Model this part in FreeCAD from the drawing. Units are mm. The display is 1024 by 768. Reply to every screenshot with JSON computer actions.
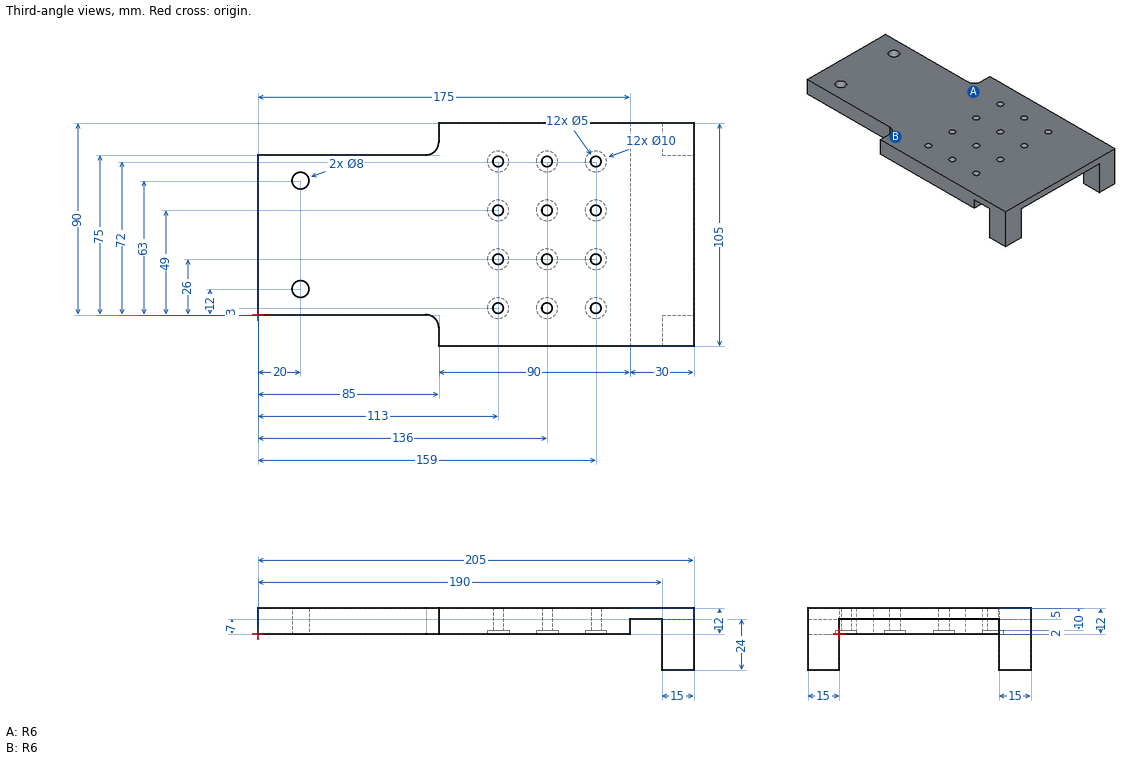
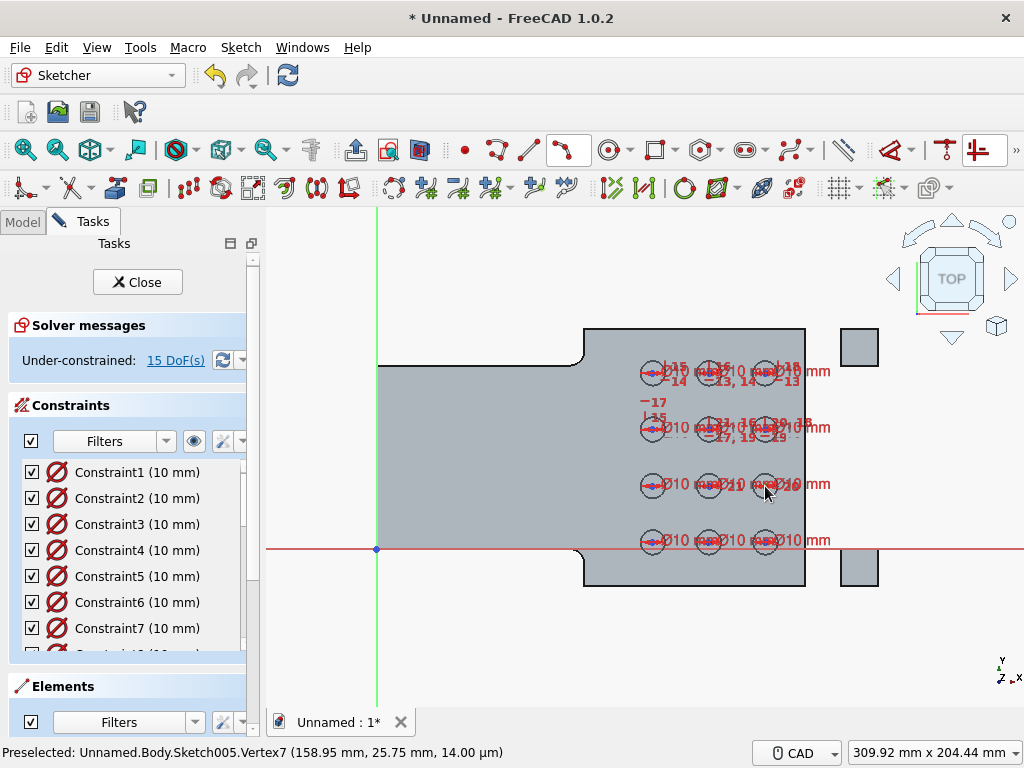
{"action": "left_click", "coordinate": [709, 486]}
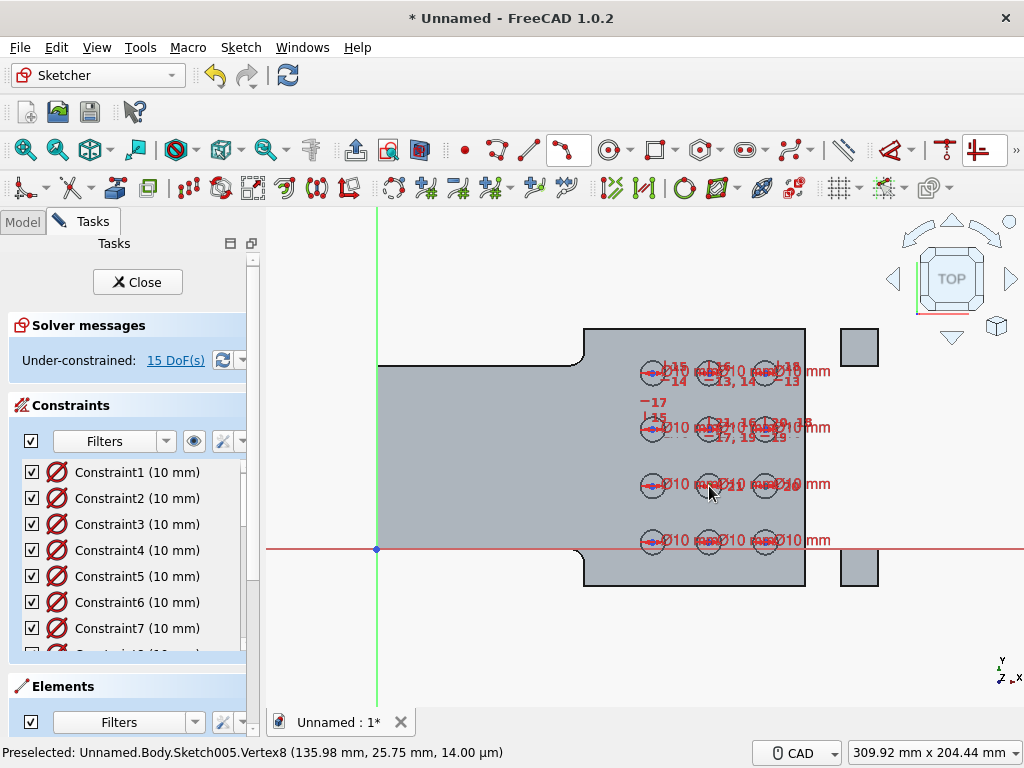
{"action": "left_click", "coordinate": [1002, 150]}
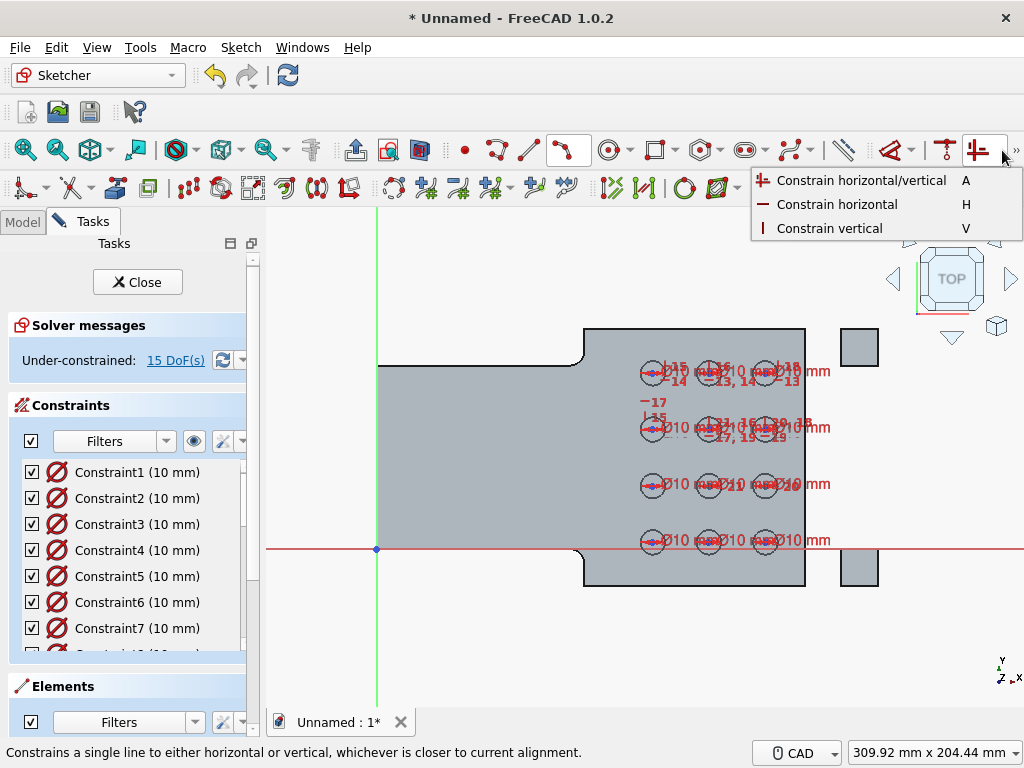
{"action": "left_click", "coordinate": [887, 204]}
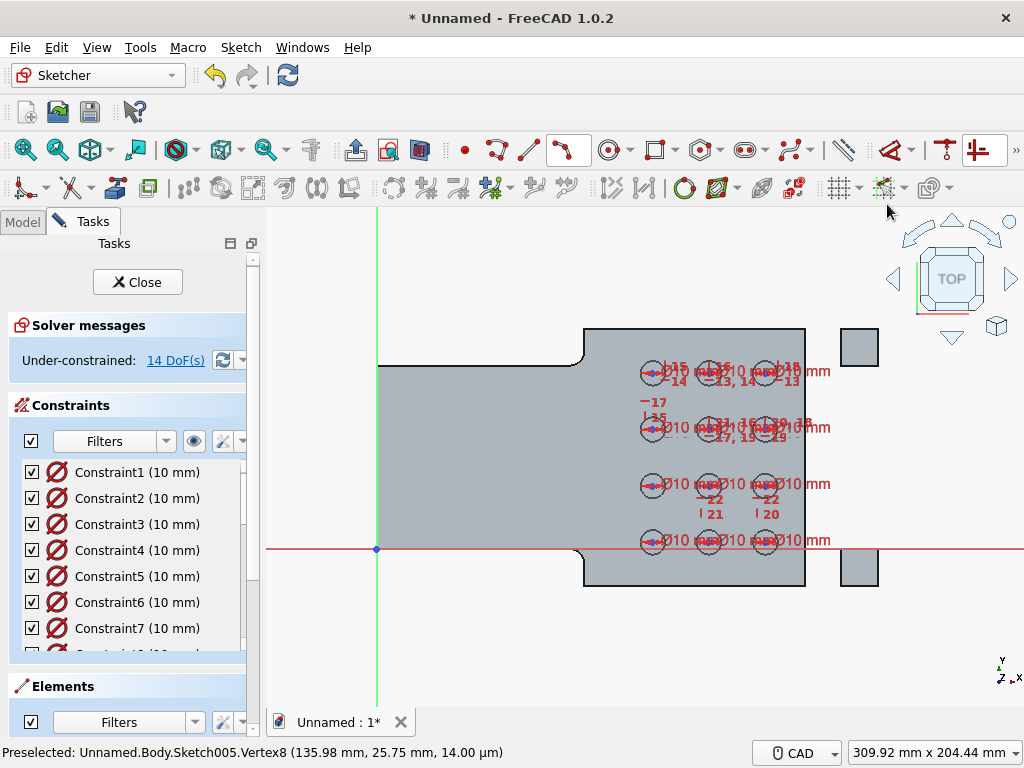
{"action": "left_click", "coordinate": [653, 430]}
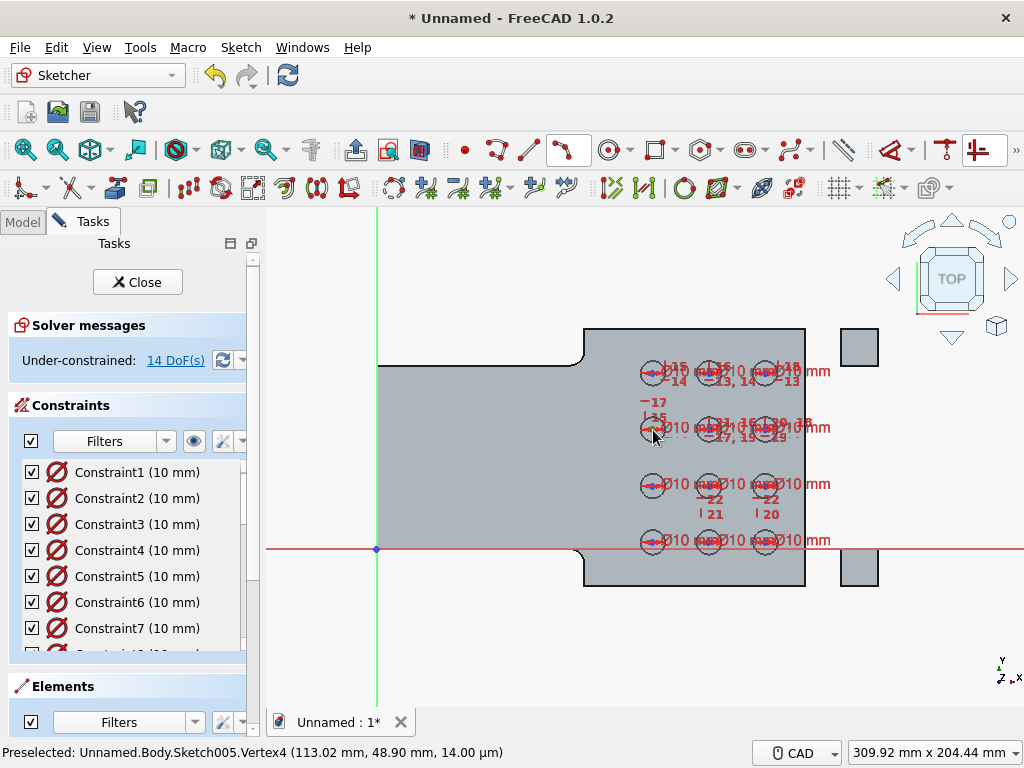
{"action": "left_click", "coordinate": [653, 486]}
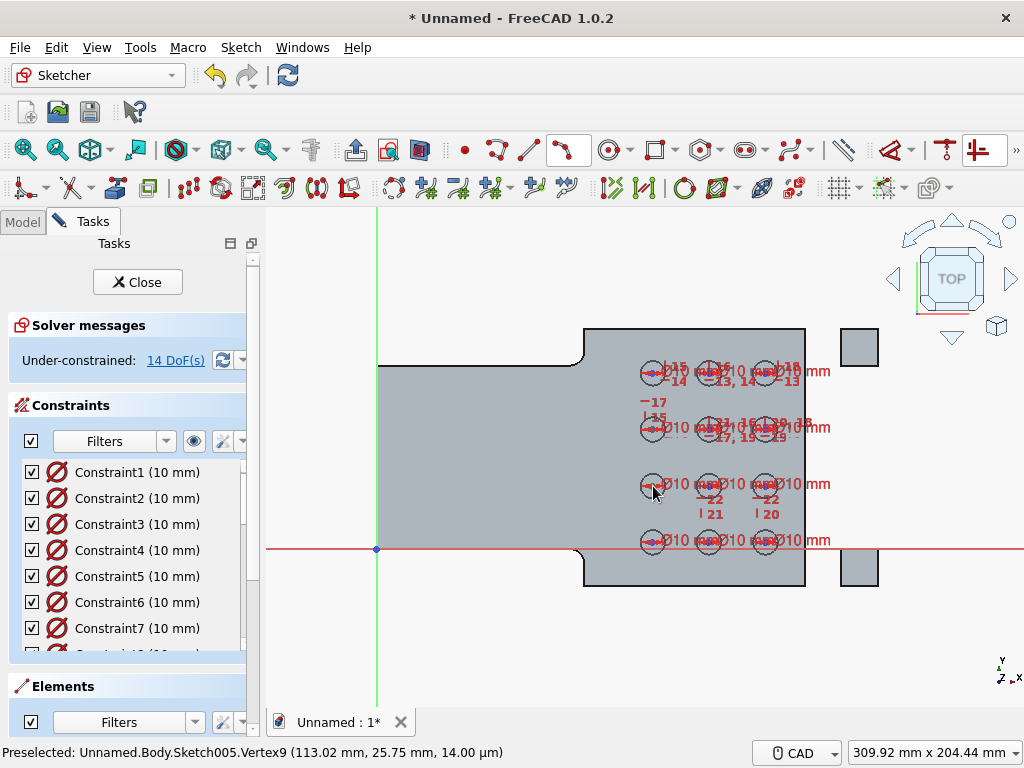
{"action": "key", "text": "v"}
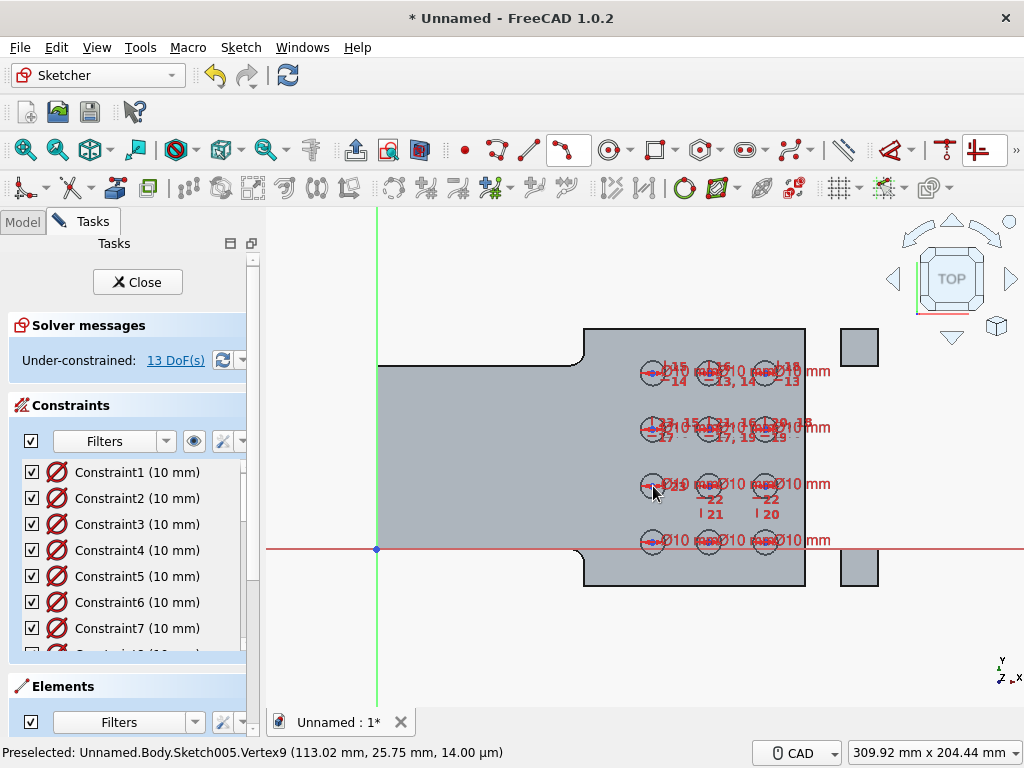
{"action": "left_click", "coordinate": [709, 486]}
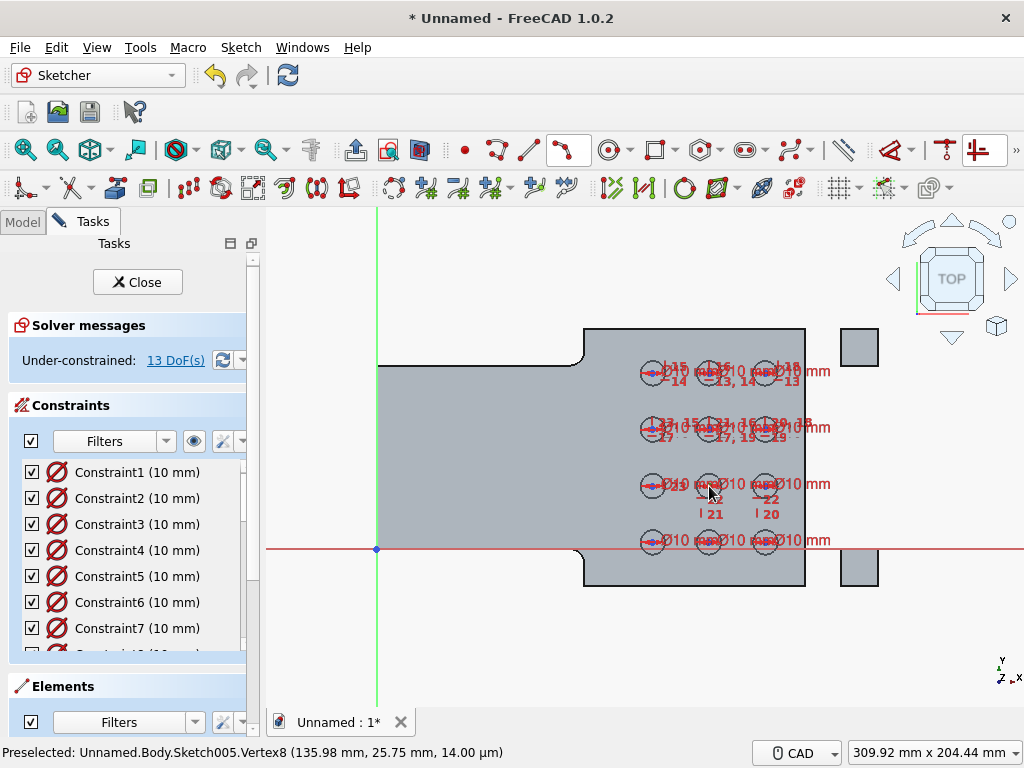
{"action": "left_click", "coordinate": [653, 486]}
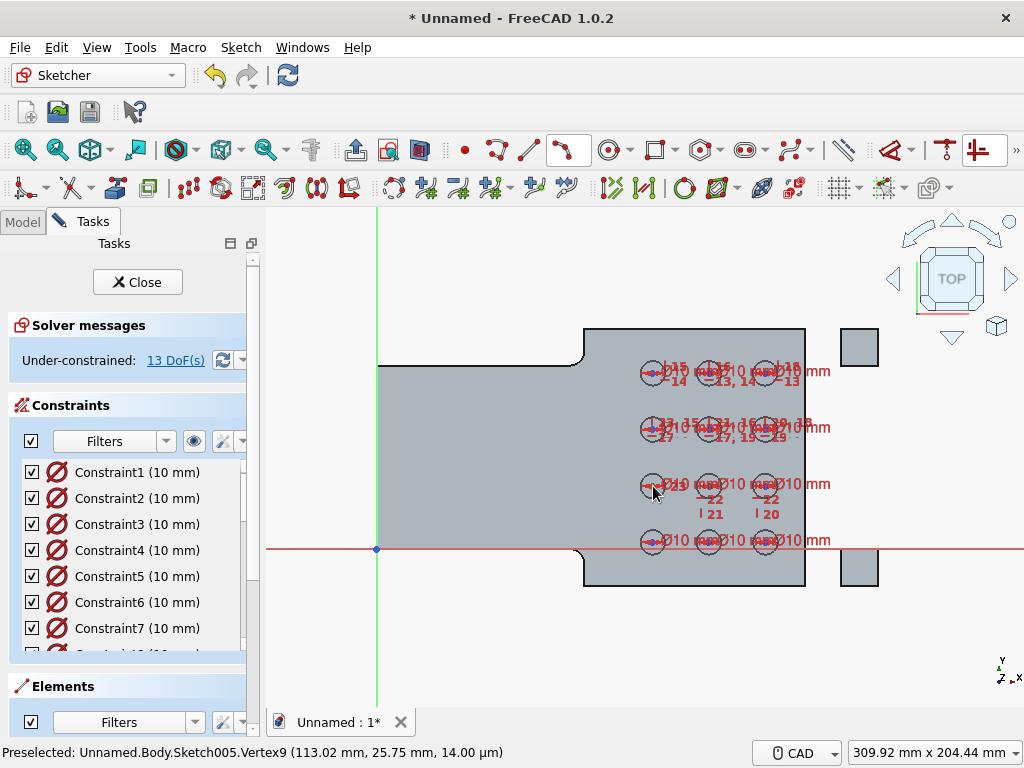
{"action": "key", "text": "h"}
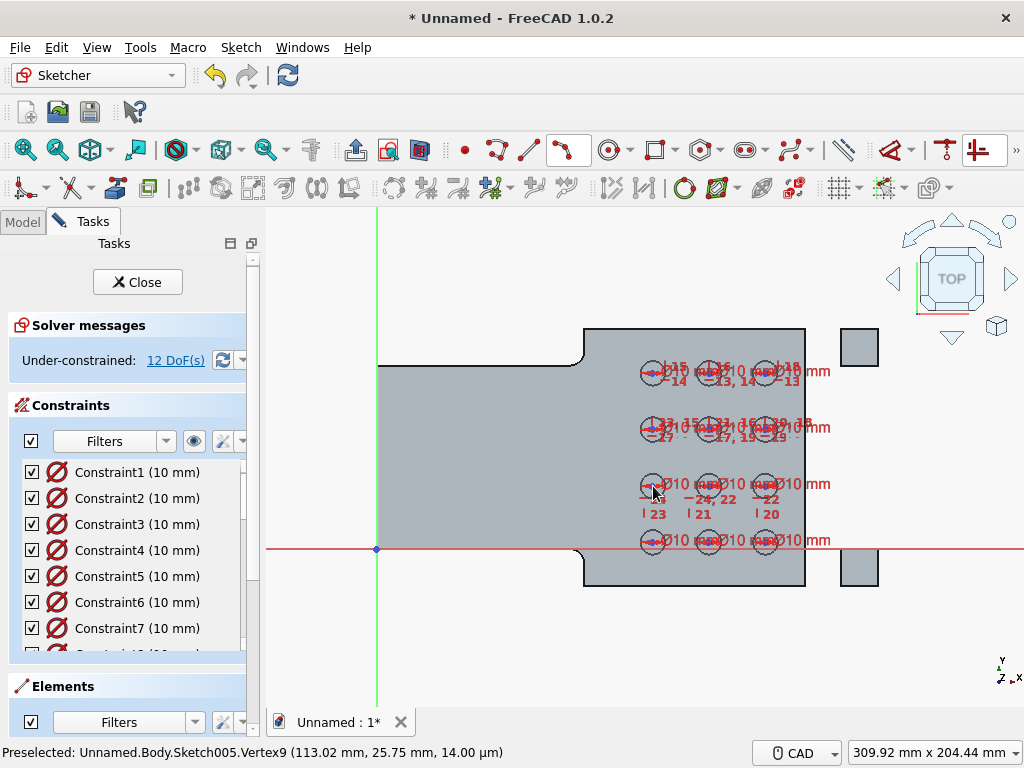
{"action": "left_click", "coordinate": [653, 486]}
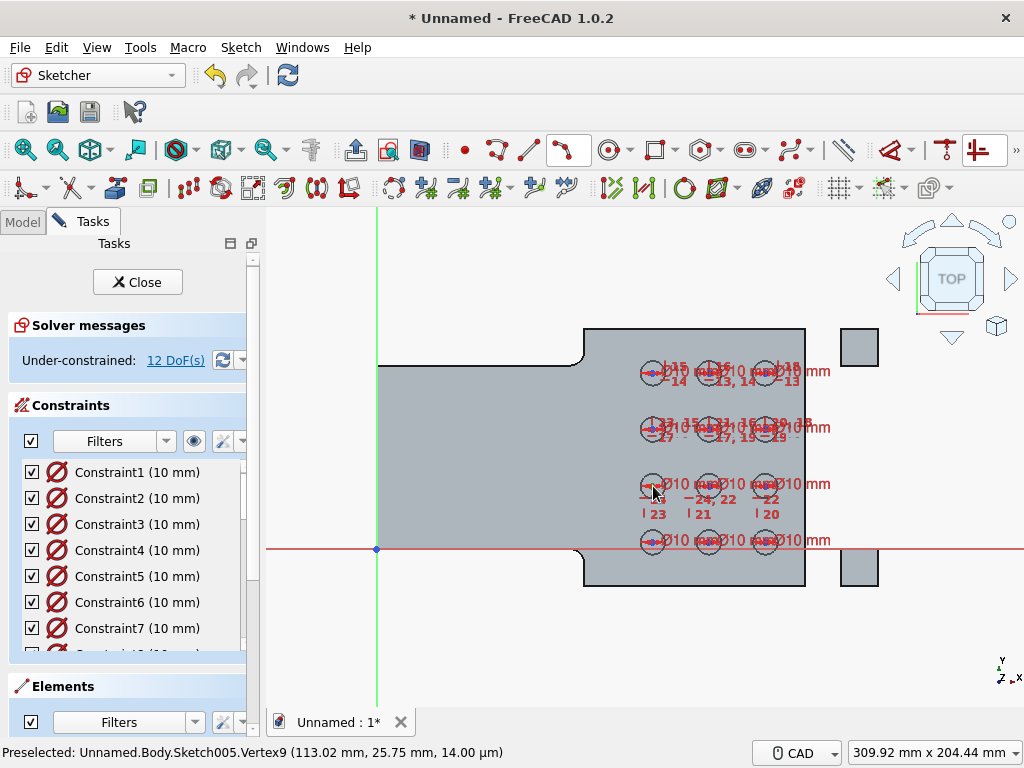
{"action": "left_click", "coordinate": [653, 542]}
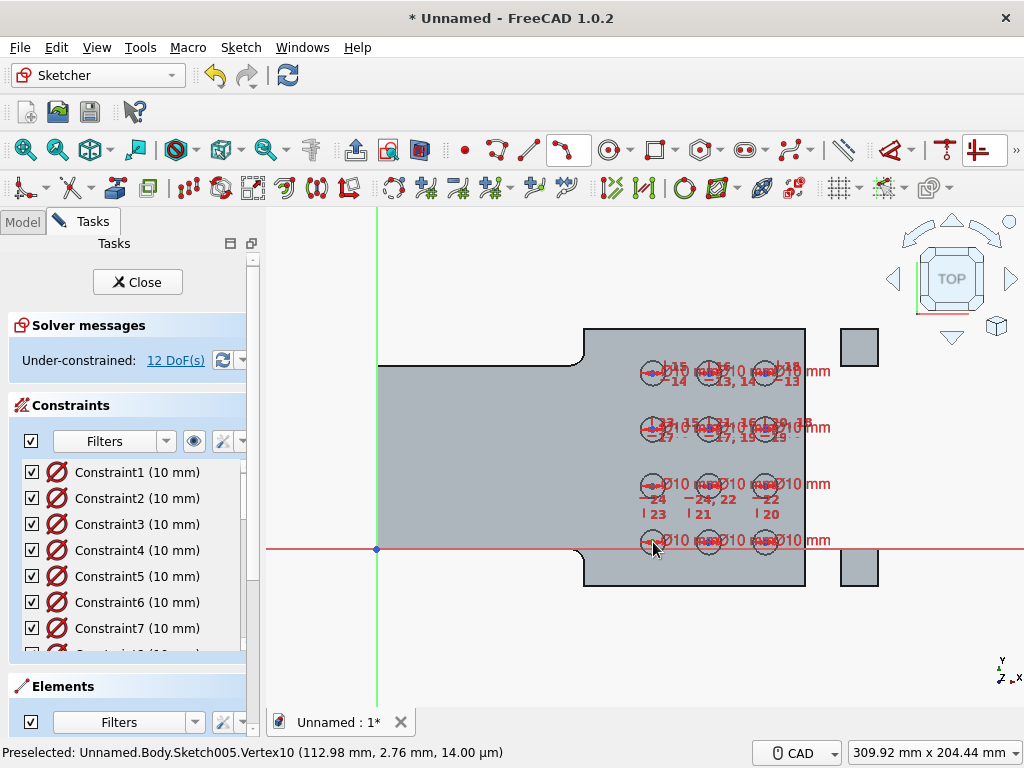
{"action": "left_click", "coordinate": [1002, 150]}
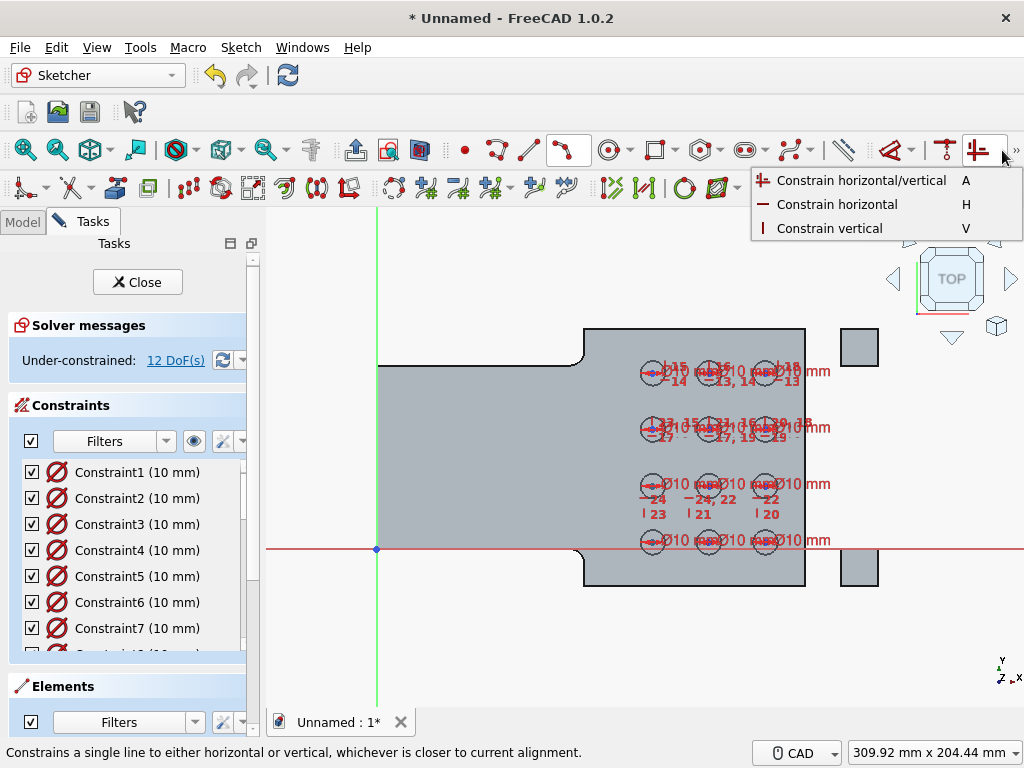
{"action": "left_click", "coordinate": [887, 228]}